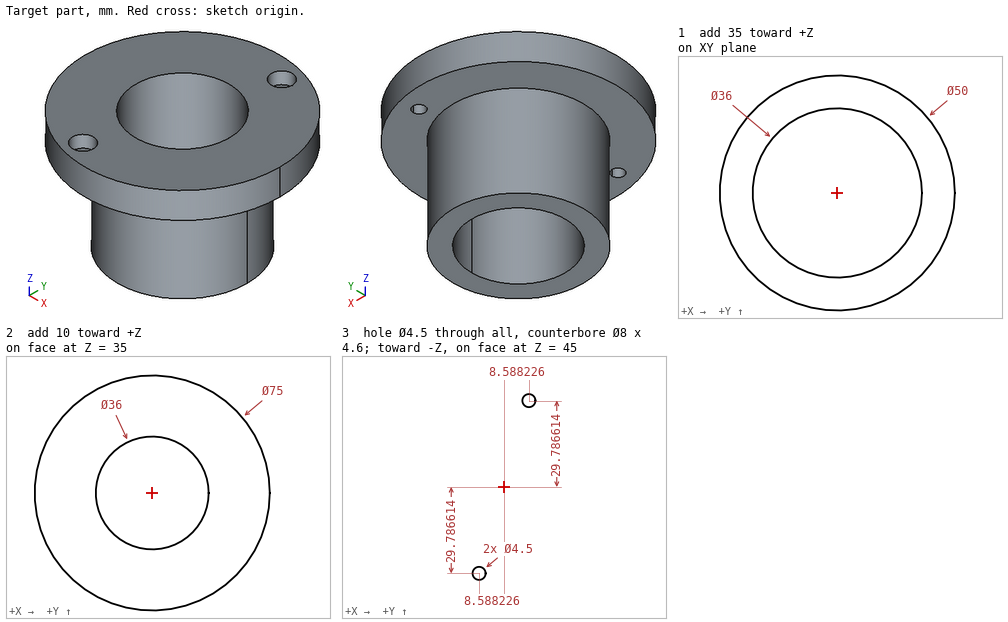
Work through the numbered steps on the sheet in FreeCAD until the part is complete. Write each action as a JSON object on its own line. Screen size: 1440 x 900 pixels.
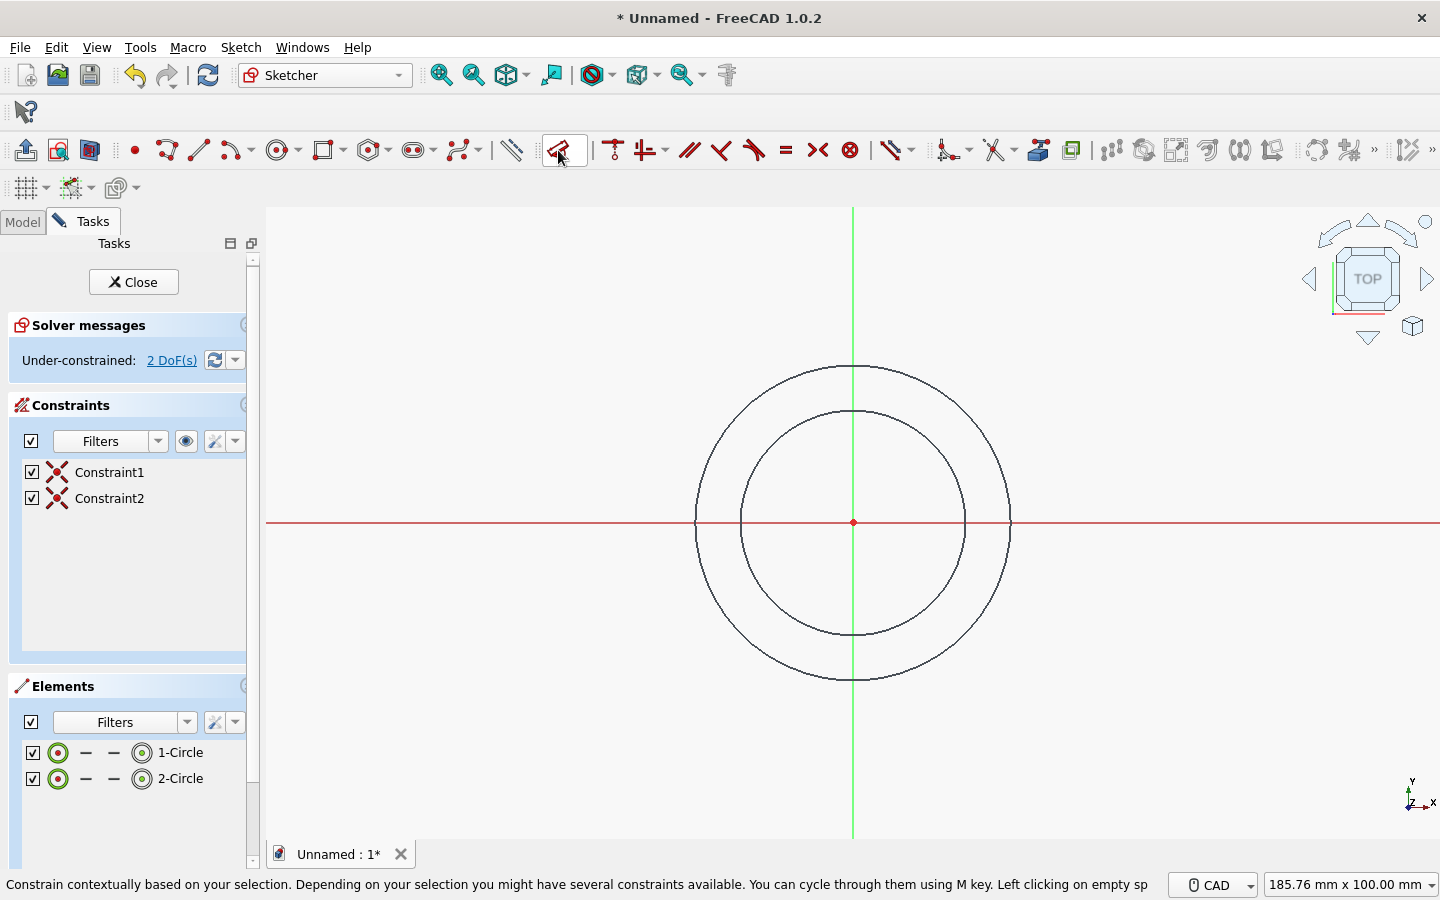
{"action": "left_click", "coordinate": [964, 411]}
{"action": "left_click", "coordinate": [987, 388]}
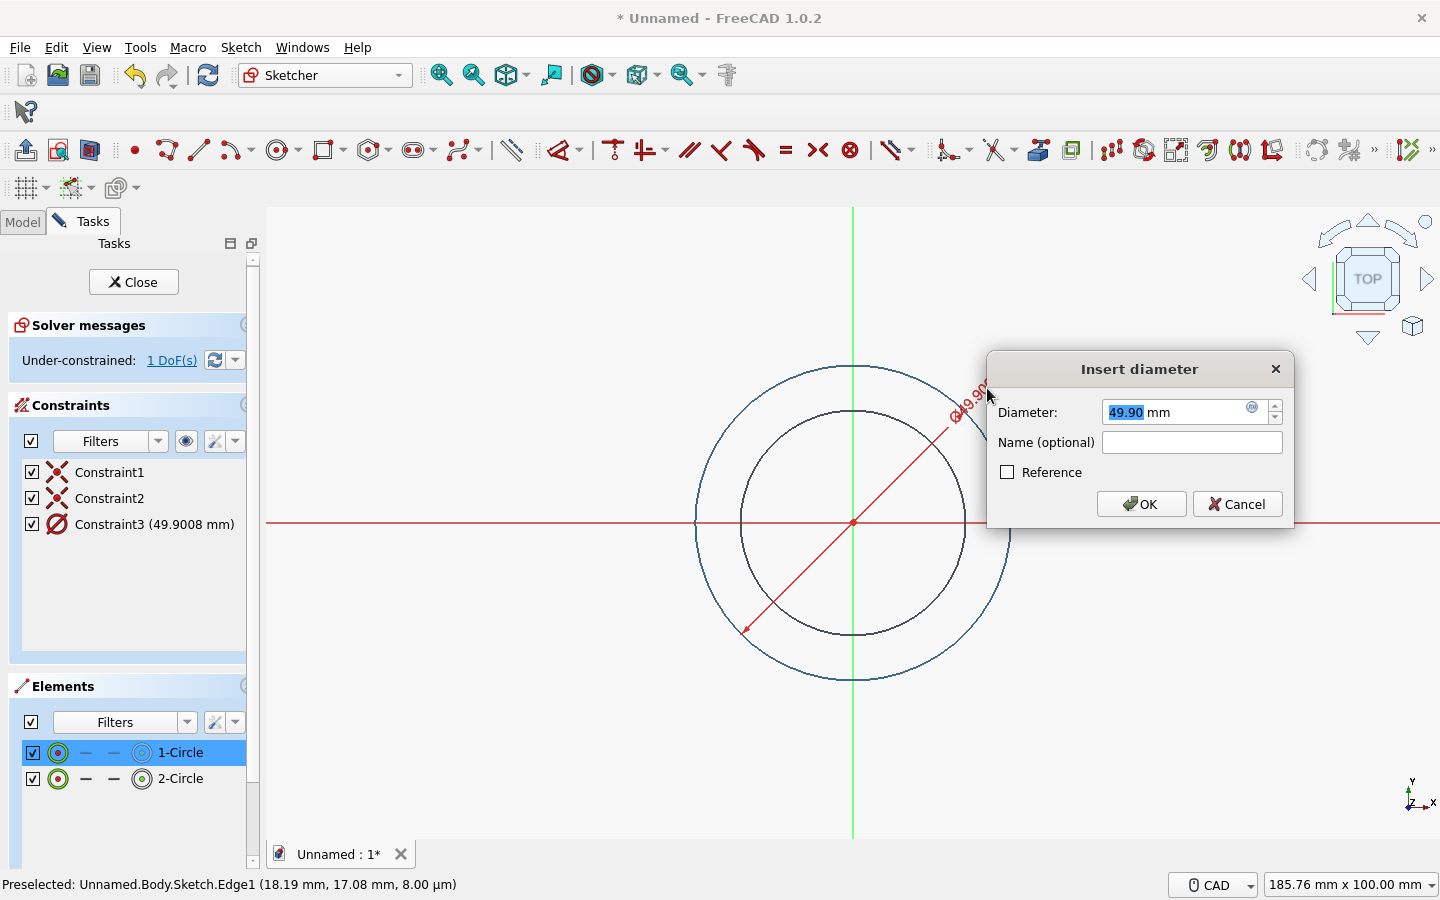
{"action": "type", "text": "50"}
{"action": "key", "text": "Return"}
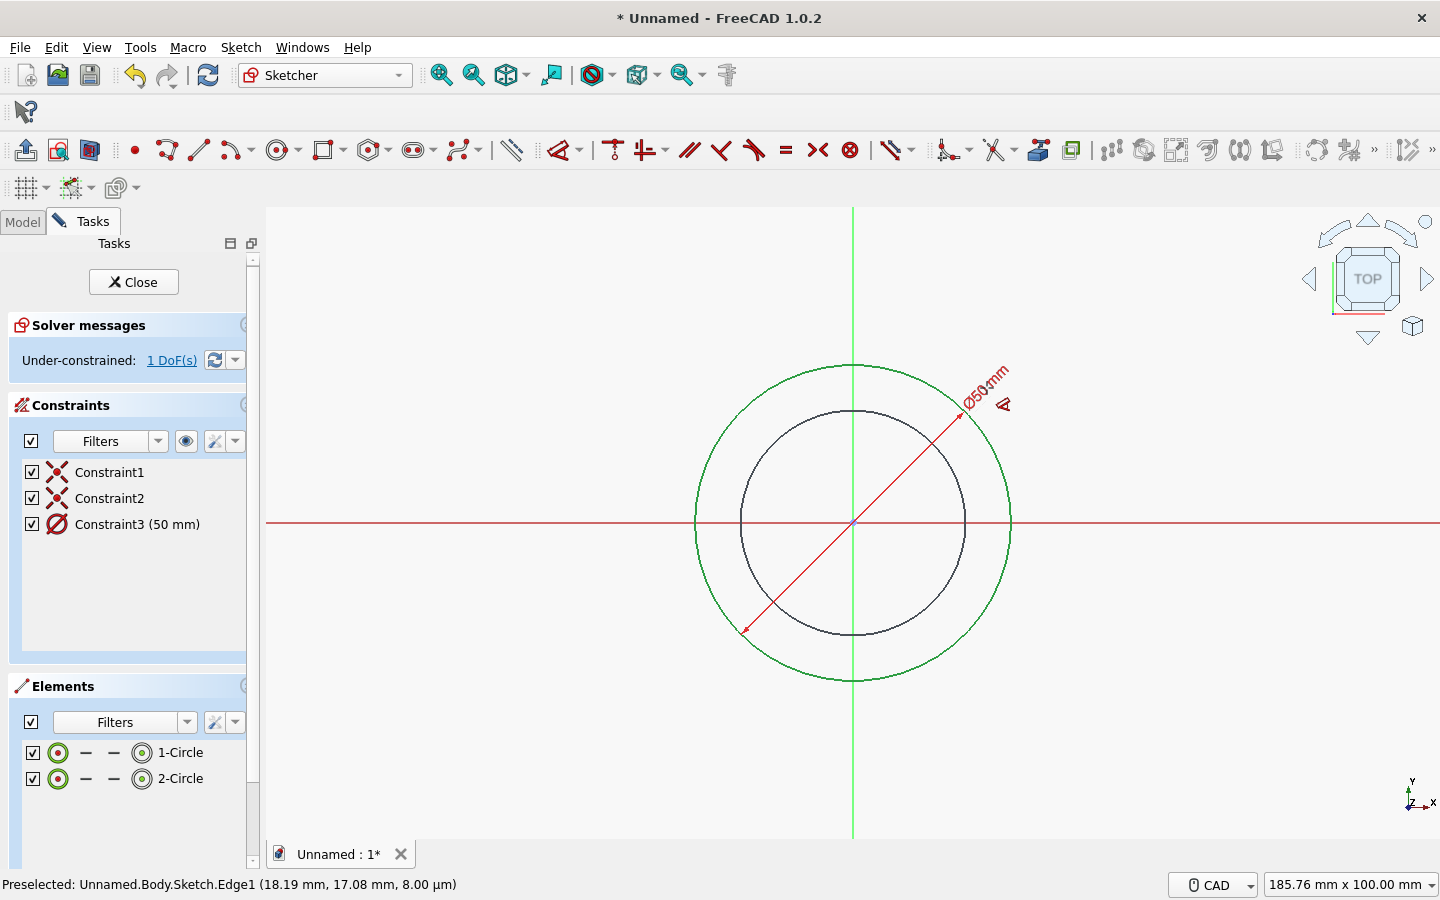
{"action": "left_click", "coordinate": [932, 443]}
{"action": "left_click", "coordinate": [954, 420]}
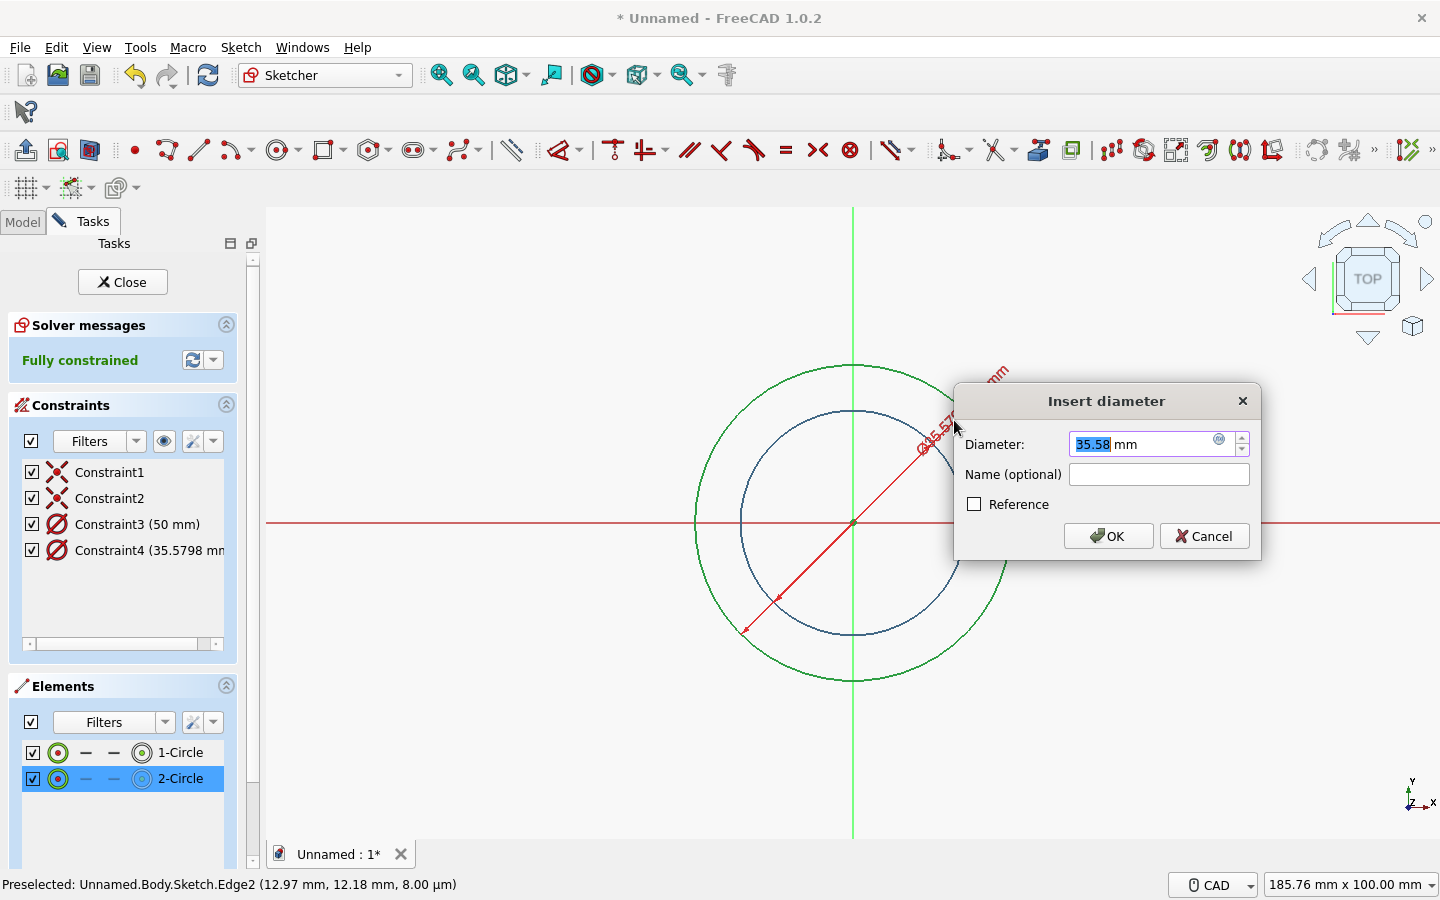
{"action": "type", "text": "36"}
{"action": "key", "text": "Return"}
{"action": "key", "text": "Escape"}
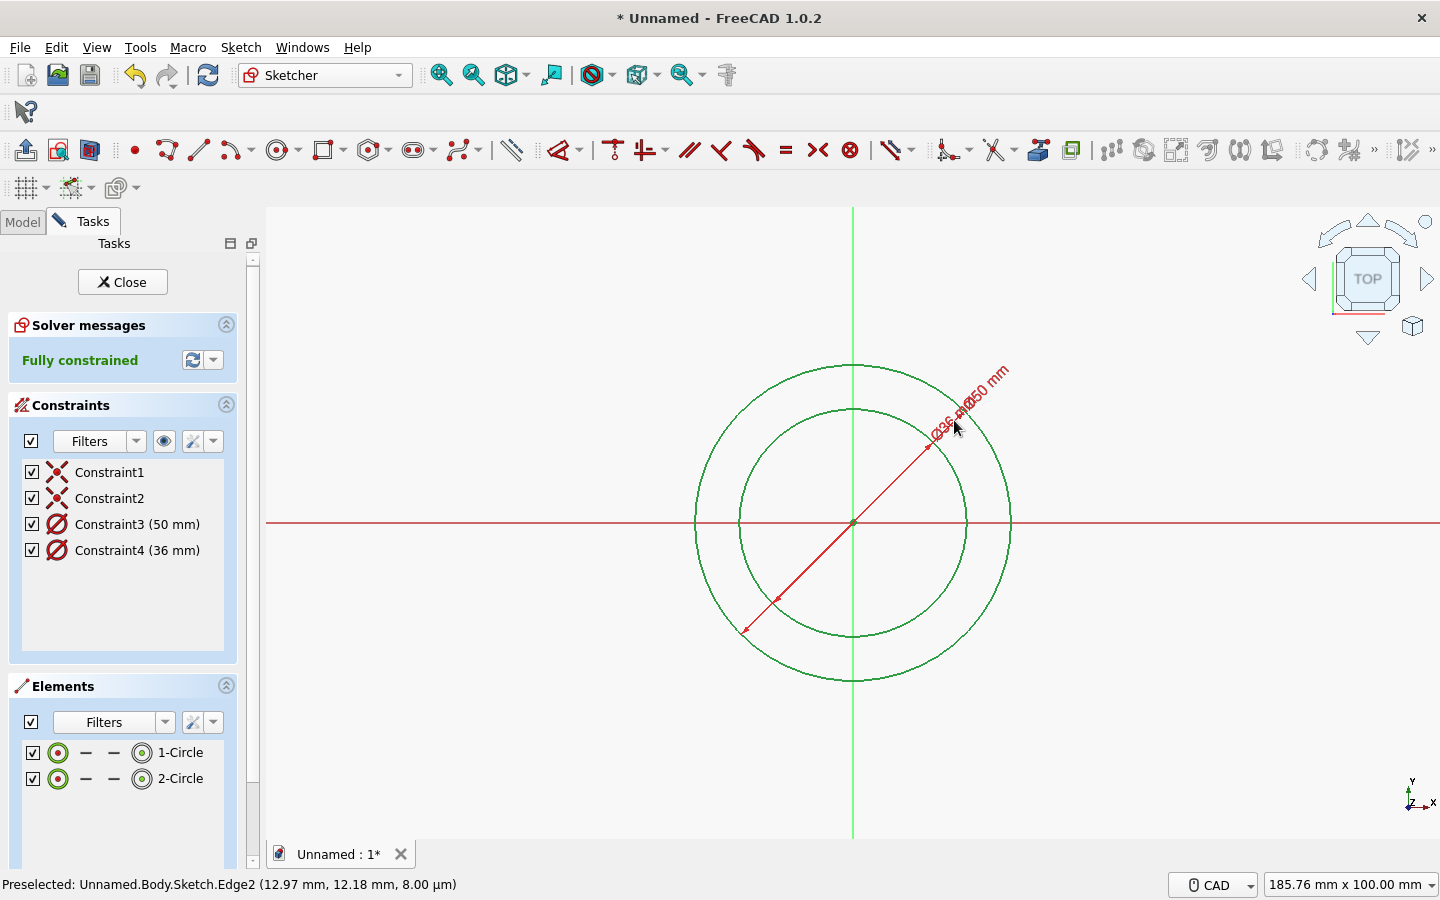
{"action": "left_click", "coordinate": [123, 282]}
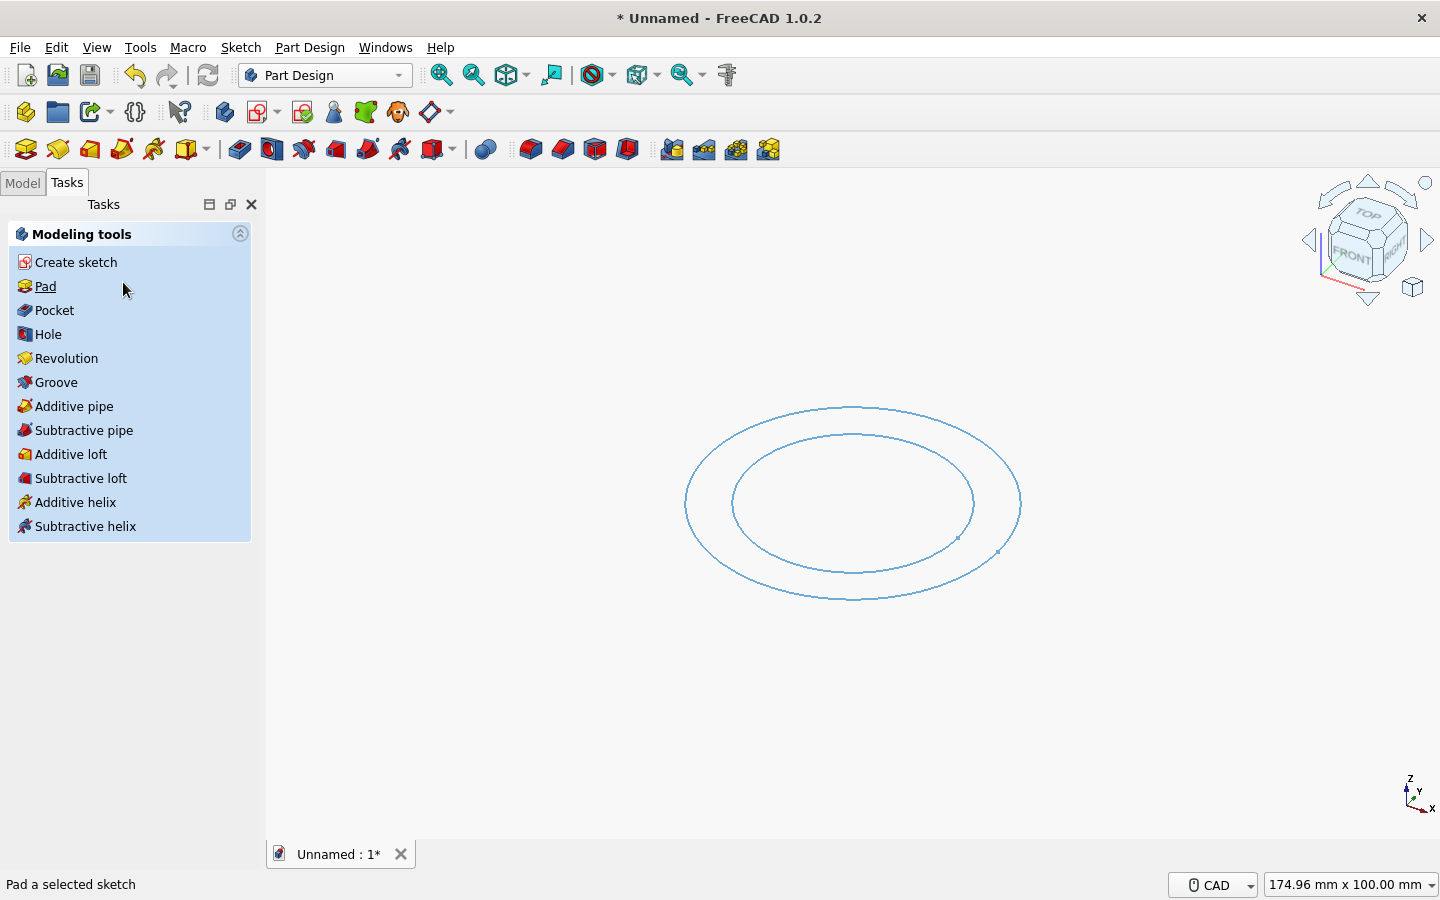
{"action": "left_click", "coordinate": [26, 150]}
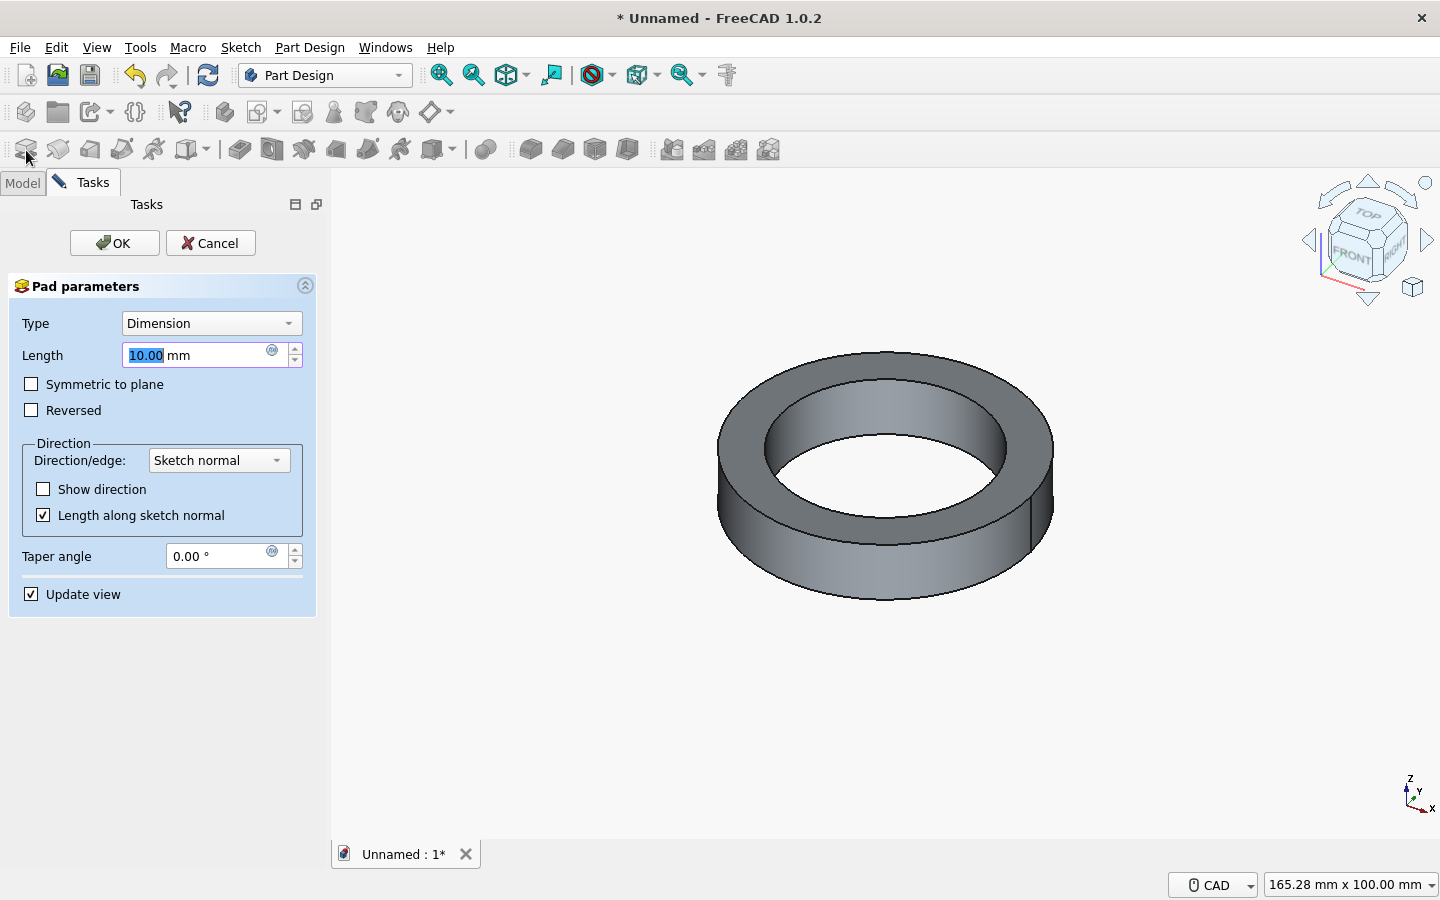
{"action": "type", "text": "35"}
{"action": "key", "text": "Tab"}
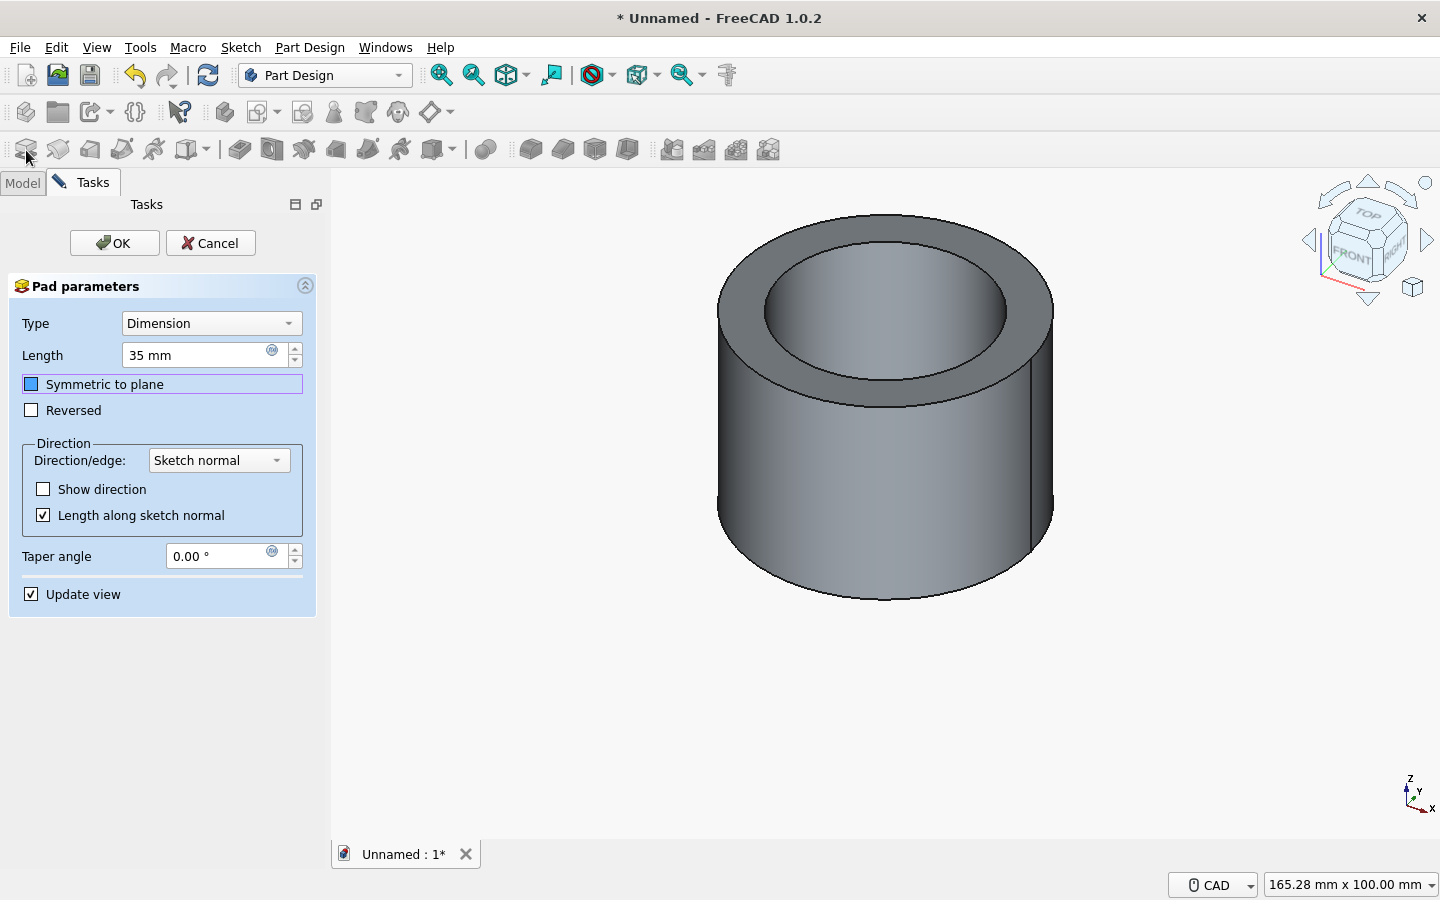
{"action": "left_click", "coordinate": [115, 243]}